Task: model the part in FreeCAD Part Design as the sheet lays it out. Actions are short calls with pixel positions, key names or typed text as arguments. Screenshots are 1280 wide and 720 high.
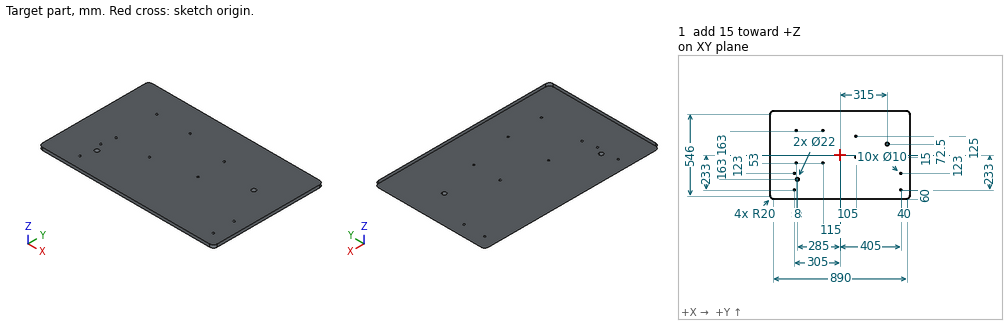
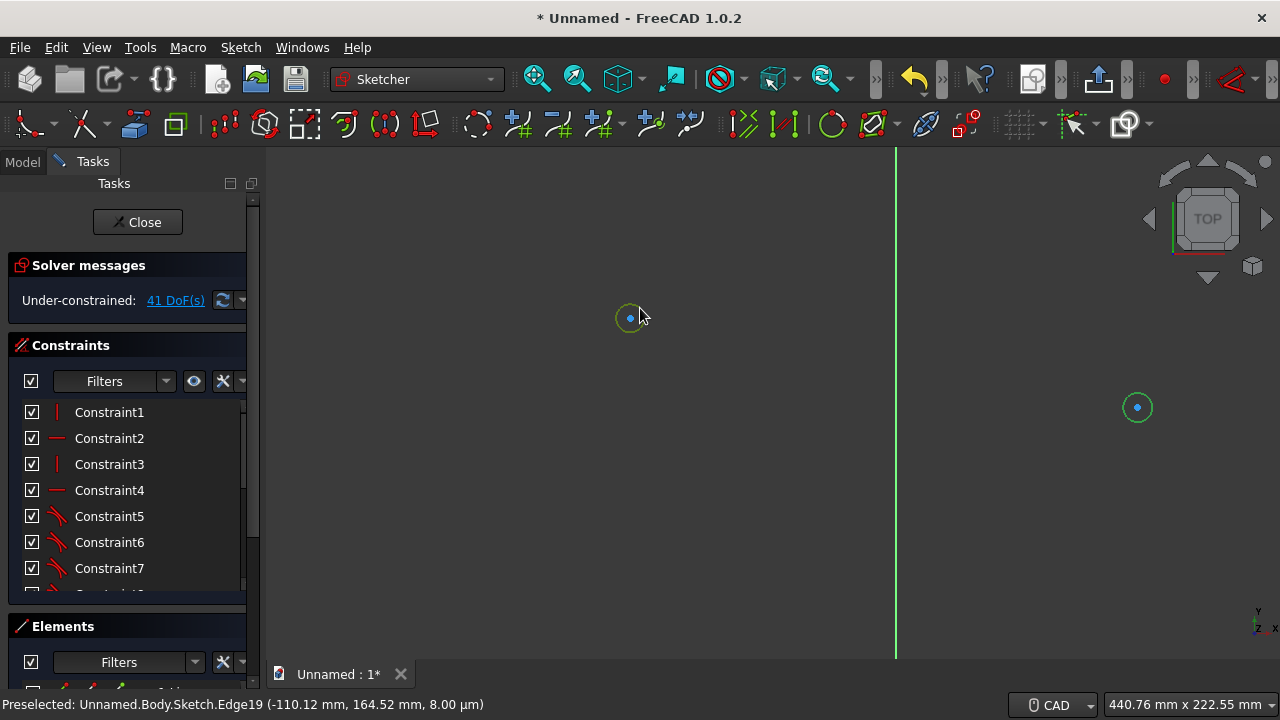
scroll(642, 309, down, 7)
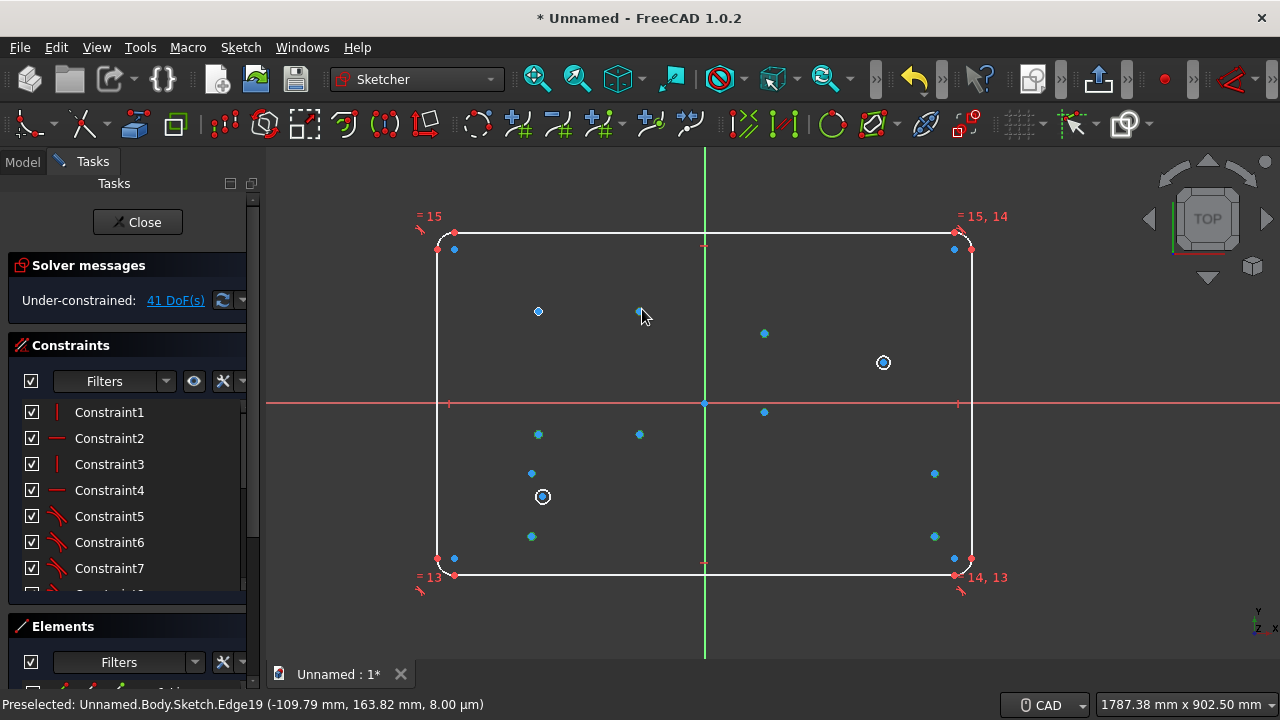
scroll(541, 309, up, 8)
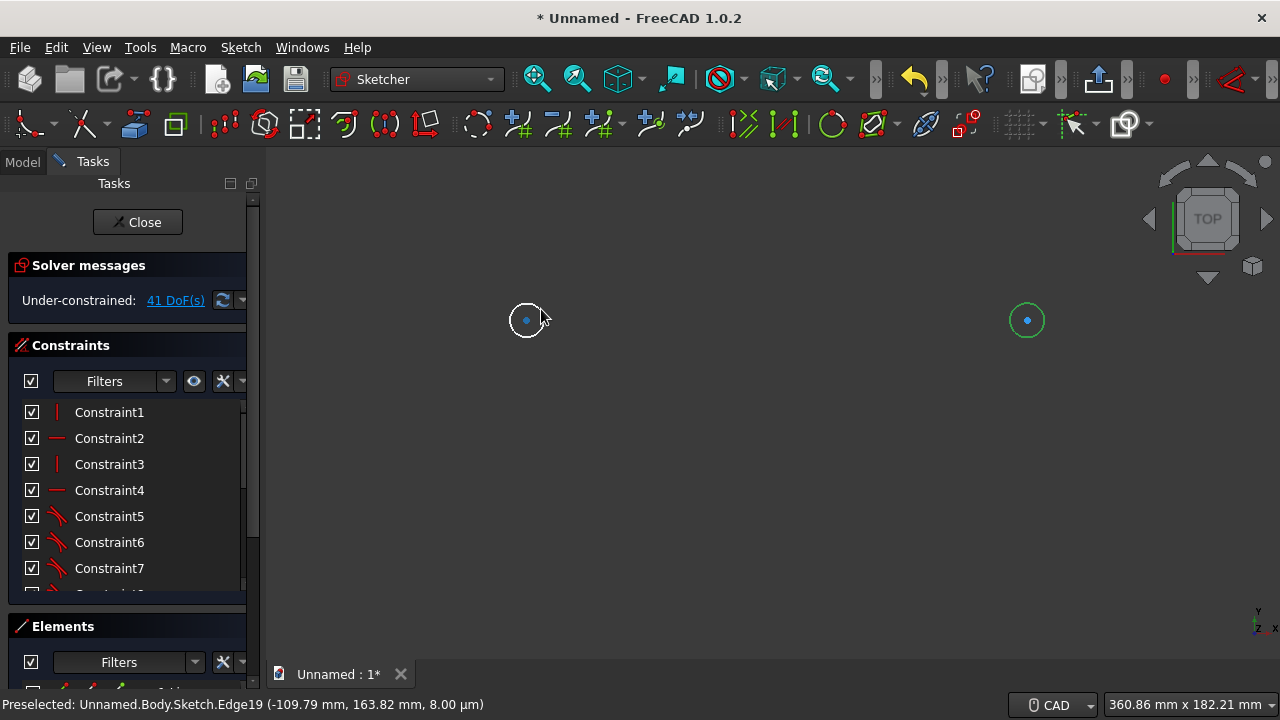
click(539, 308)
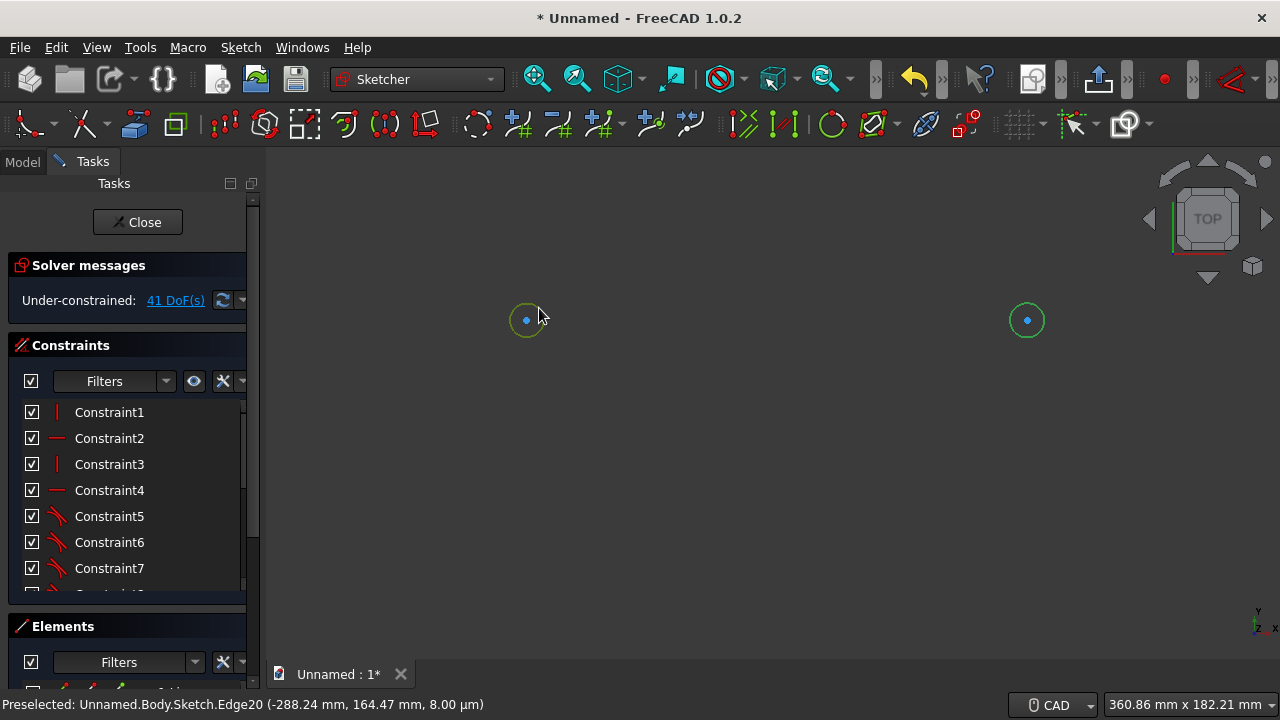
key(e)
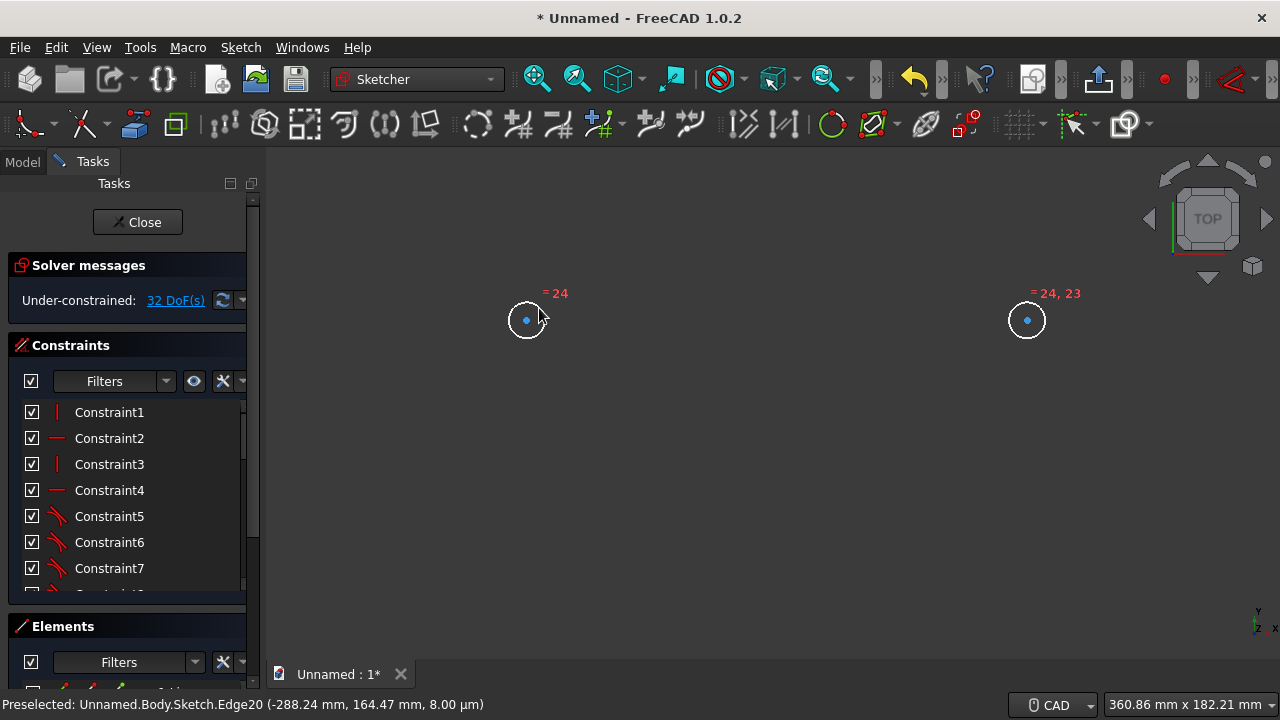
scroll(541, 309, down, 8)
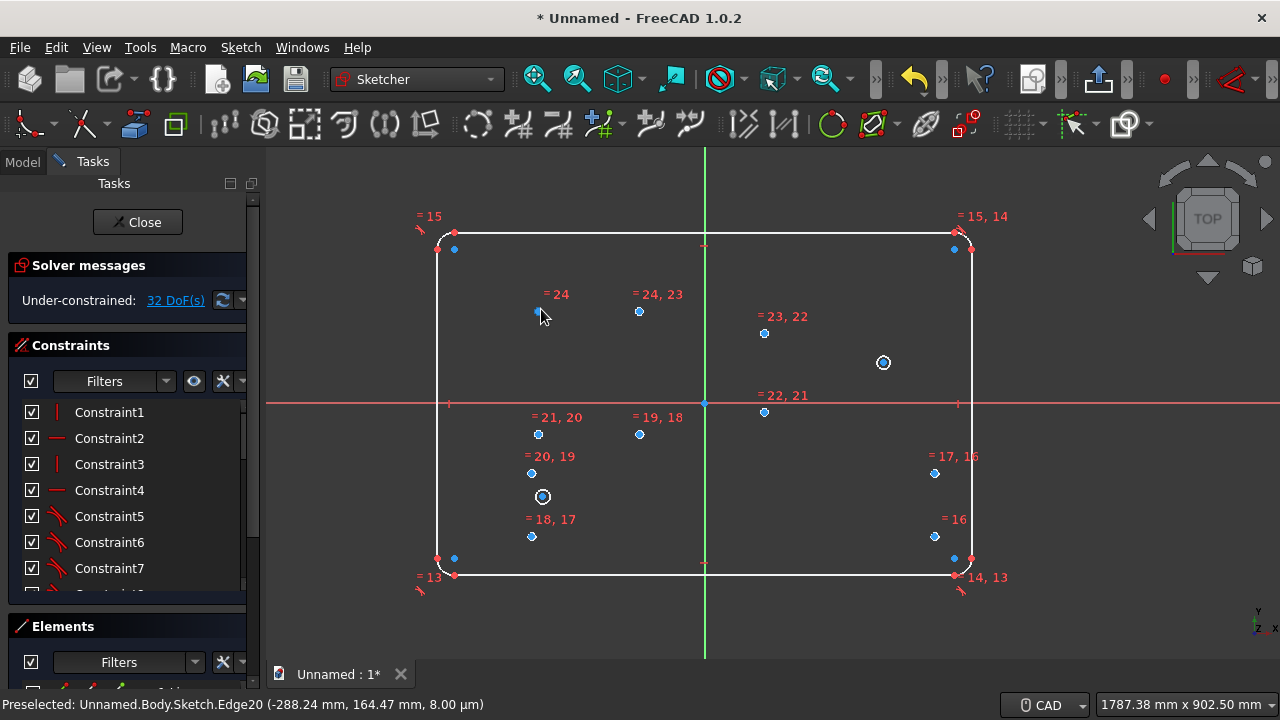
scroll(548, 492, up, 4)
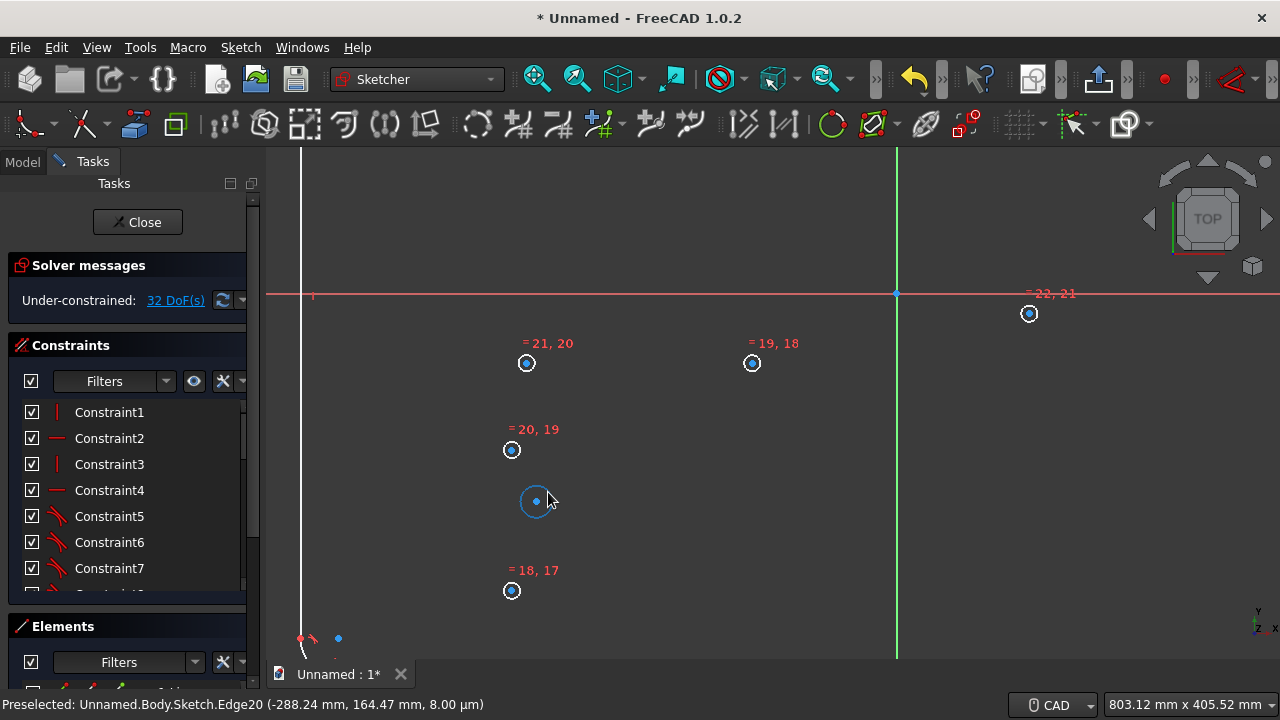
click(548, 490)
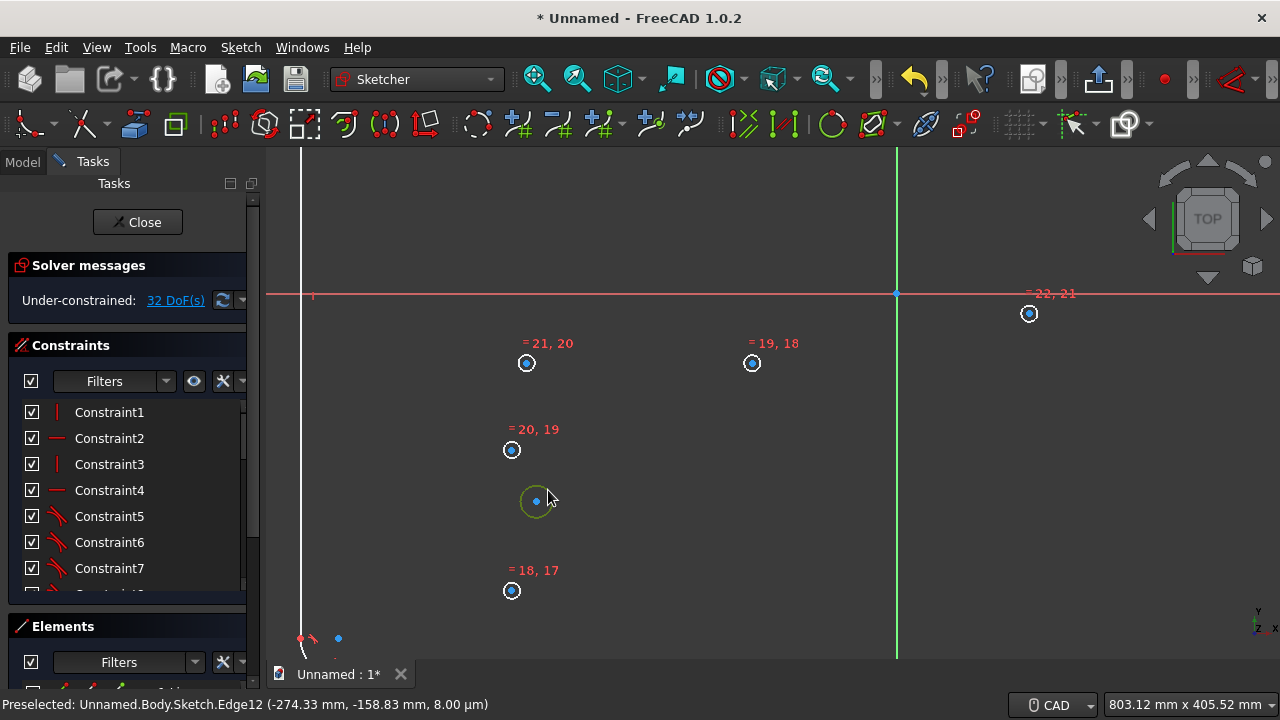
scroll(548, 492, down, 4)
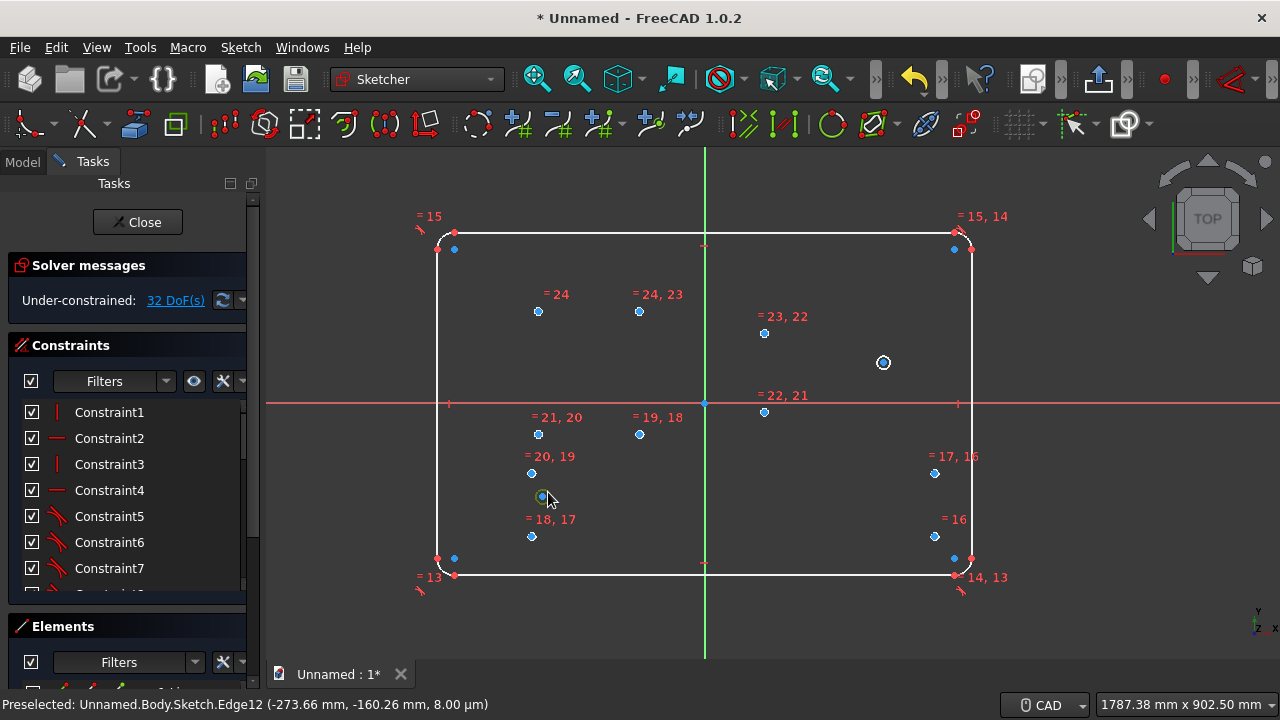
scroll(888, 358, up, 4)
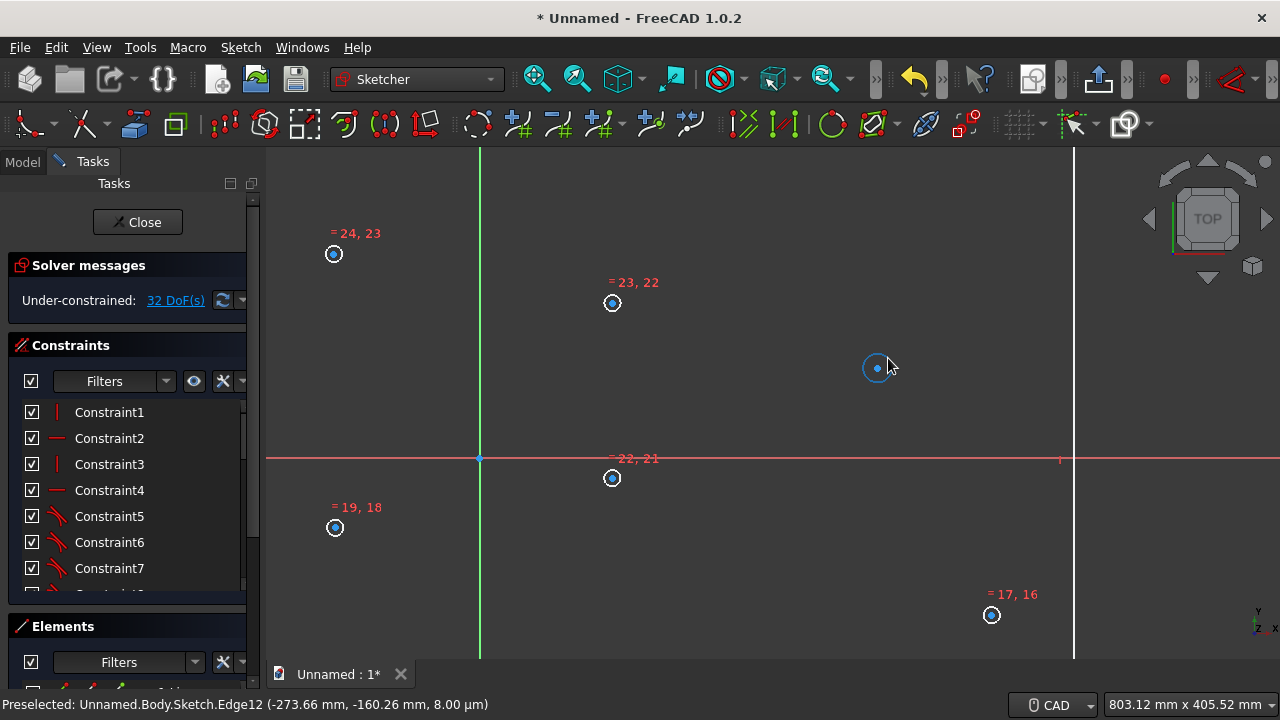
click(888, 358)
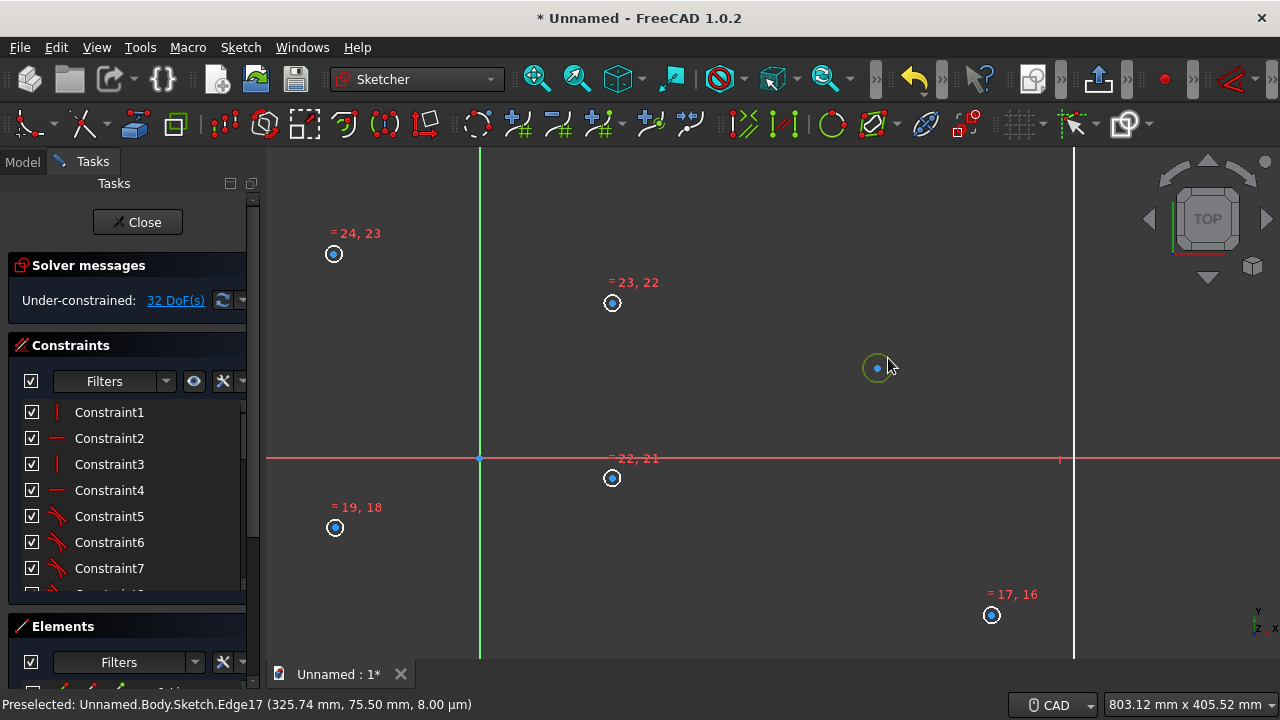
key(e)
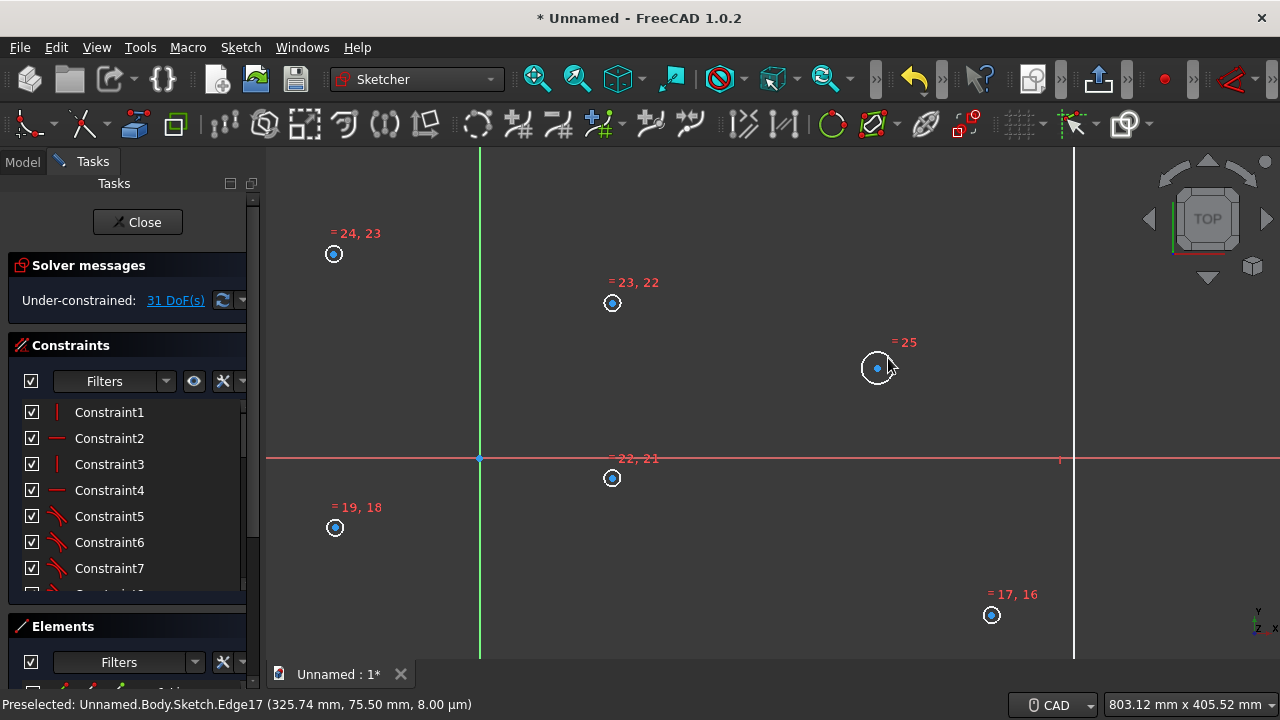
scroll(888, 358, down, 4)